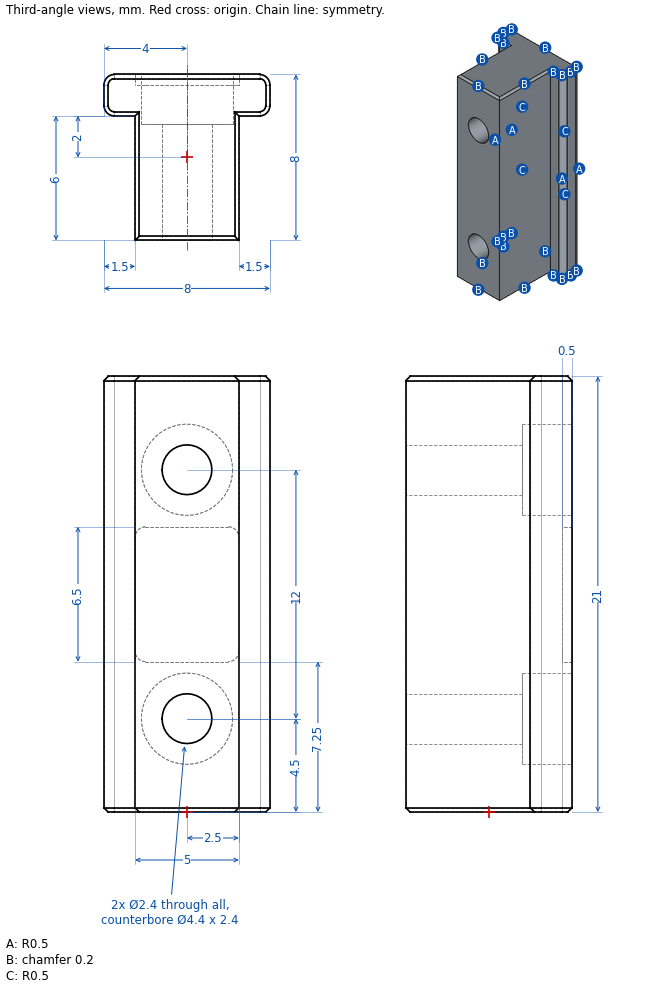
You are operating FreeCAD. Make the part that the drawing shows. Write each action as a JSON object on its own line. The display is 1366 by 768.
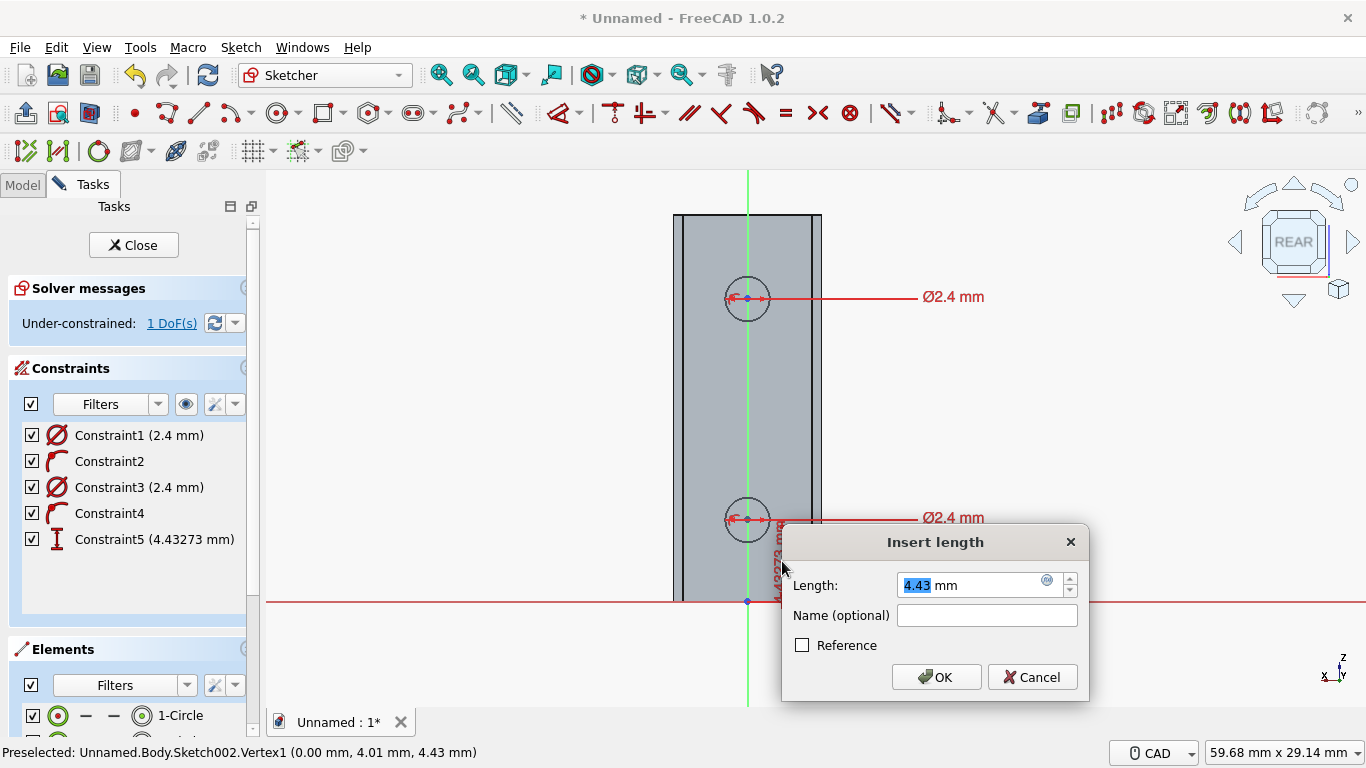
{"action": "type", "text": "4.5"}
{"action": "key", "text": "Return"}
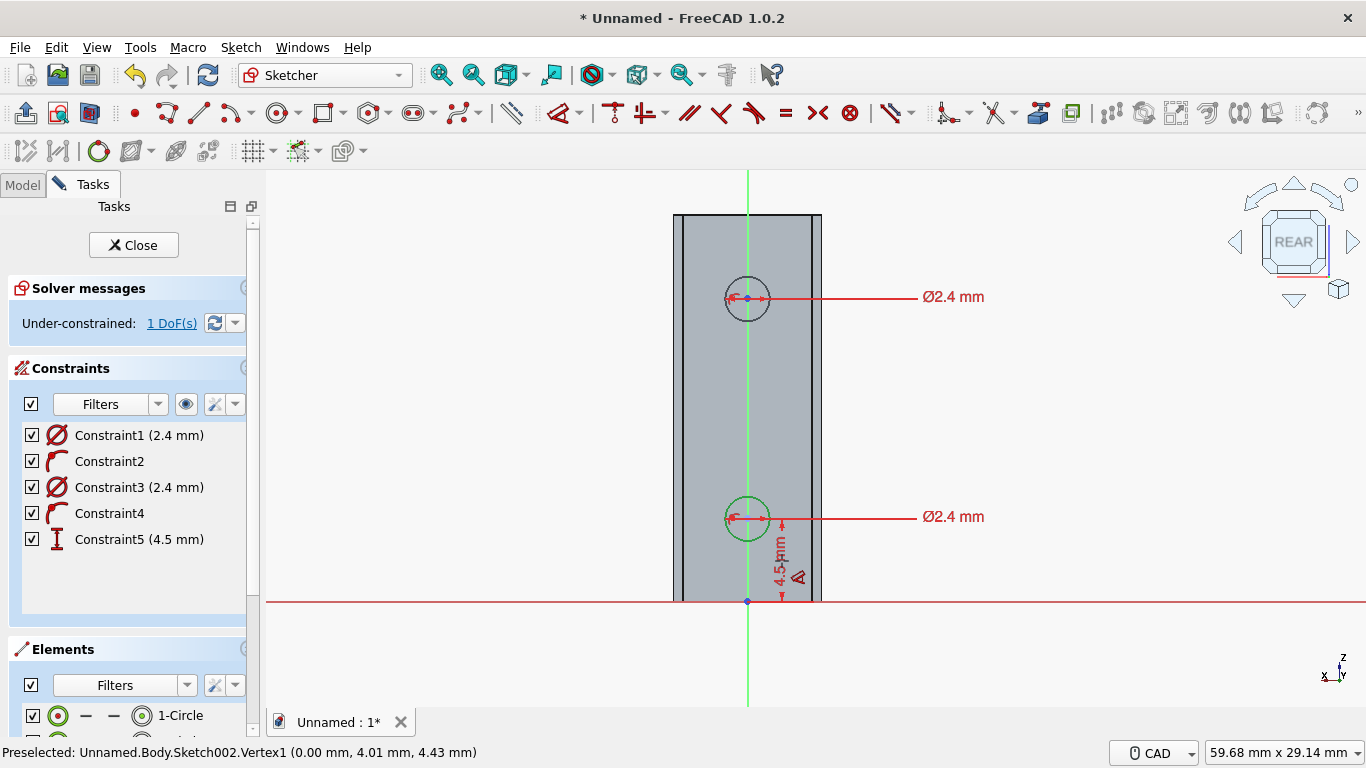
{"action": "left_click", "coordinate": [748, 519]}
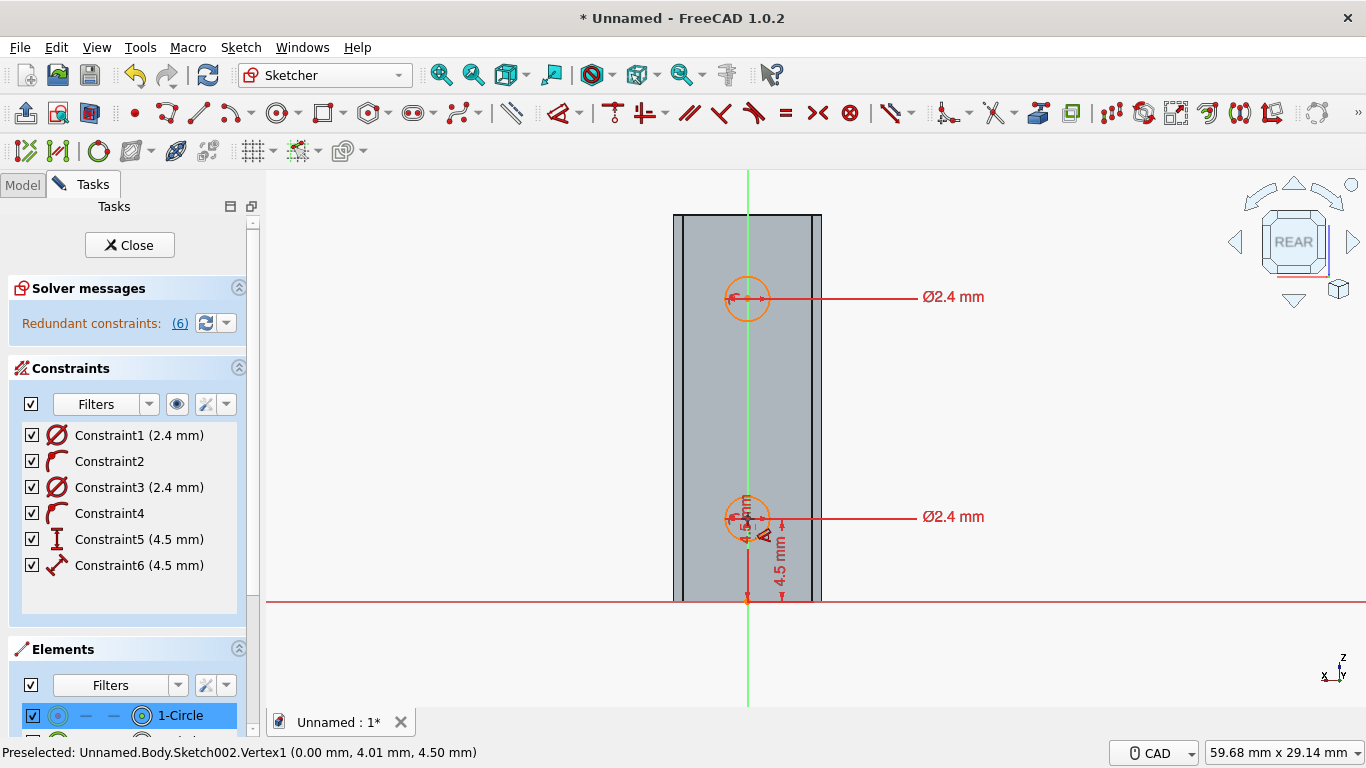
{"action": "left_click", "coordinate": [748, 299]}
{"action": "left_click", "coordinate": [782, 409]}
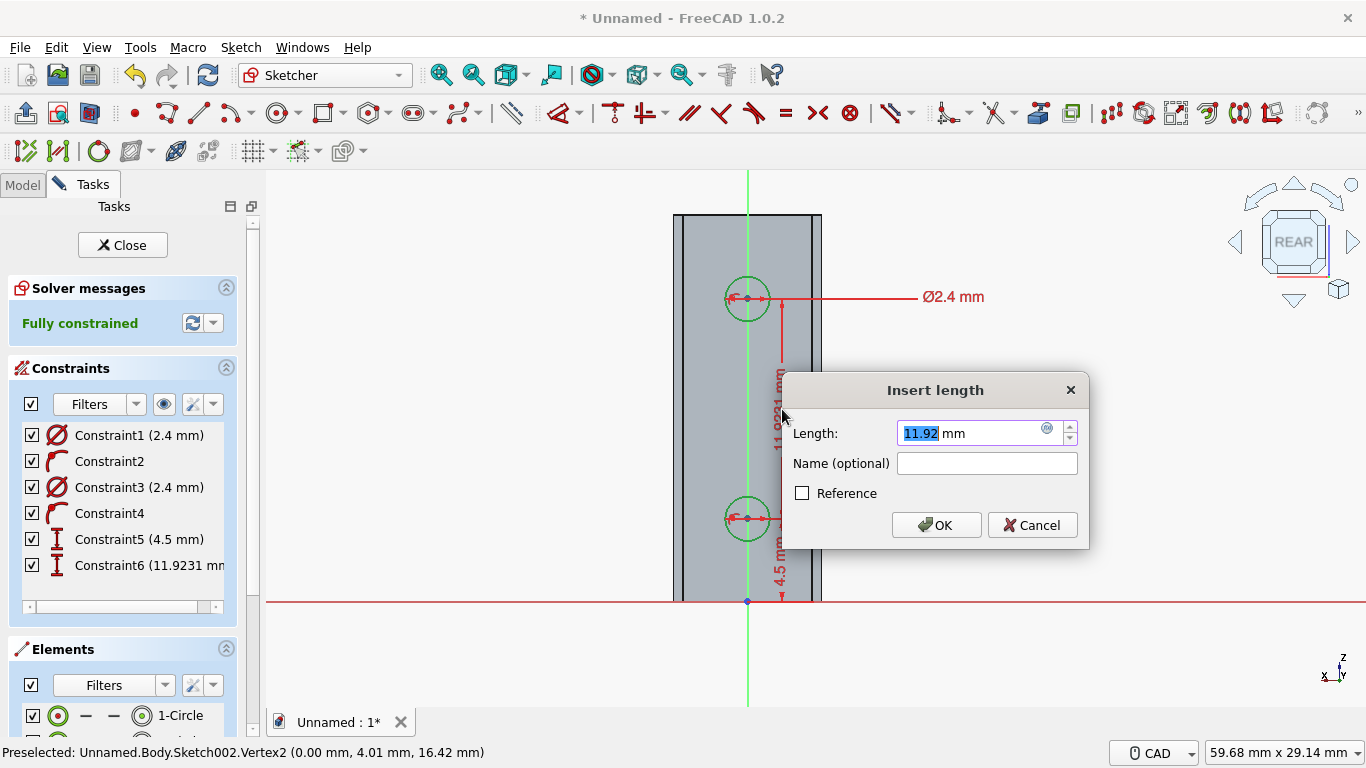
{"action": "type", "text": "12"}
{"action": "key", "text": "Return"}
{"action": "key", "text": "Escape"}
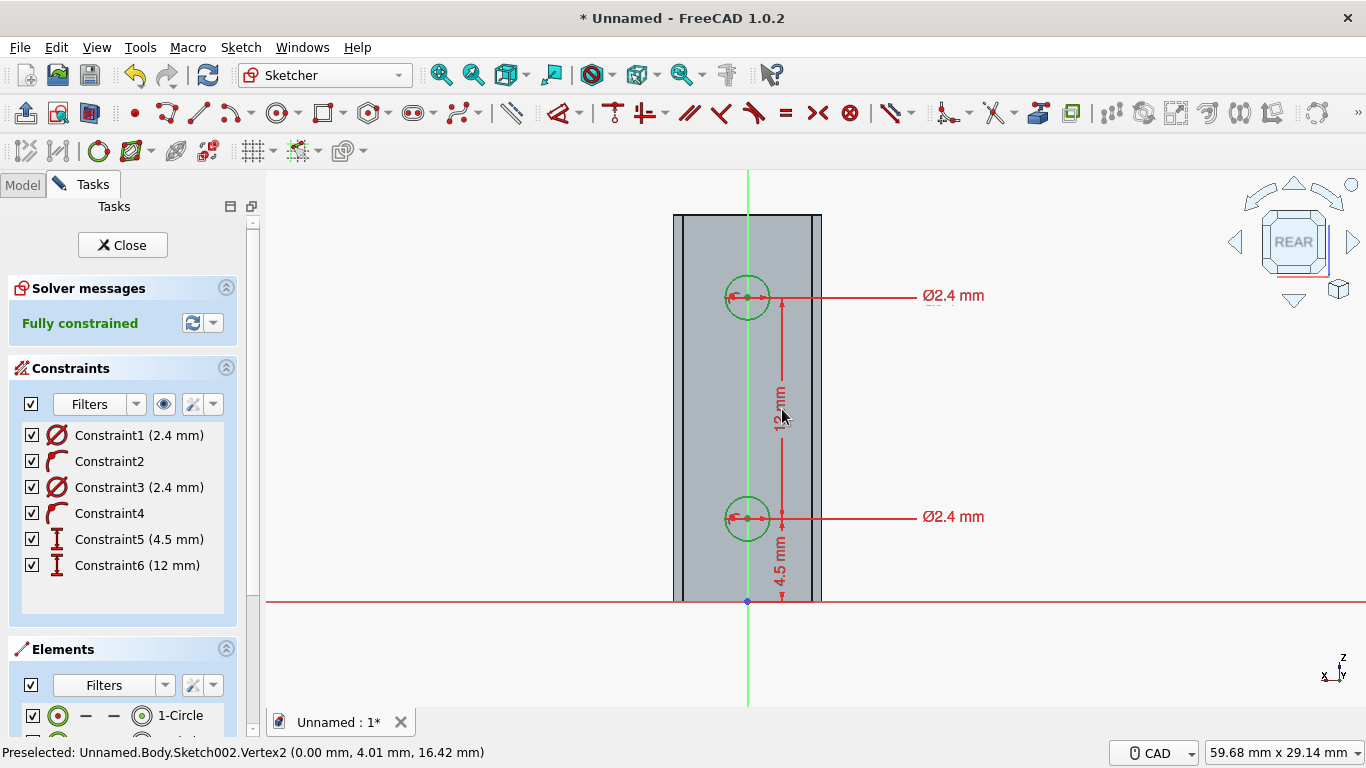
{"action": "left_click", "coordinate": [123, 245]}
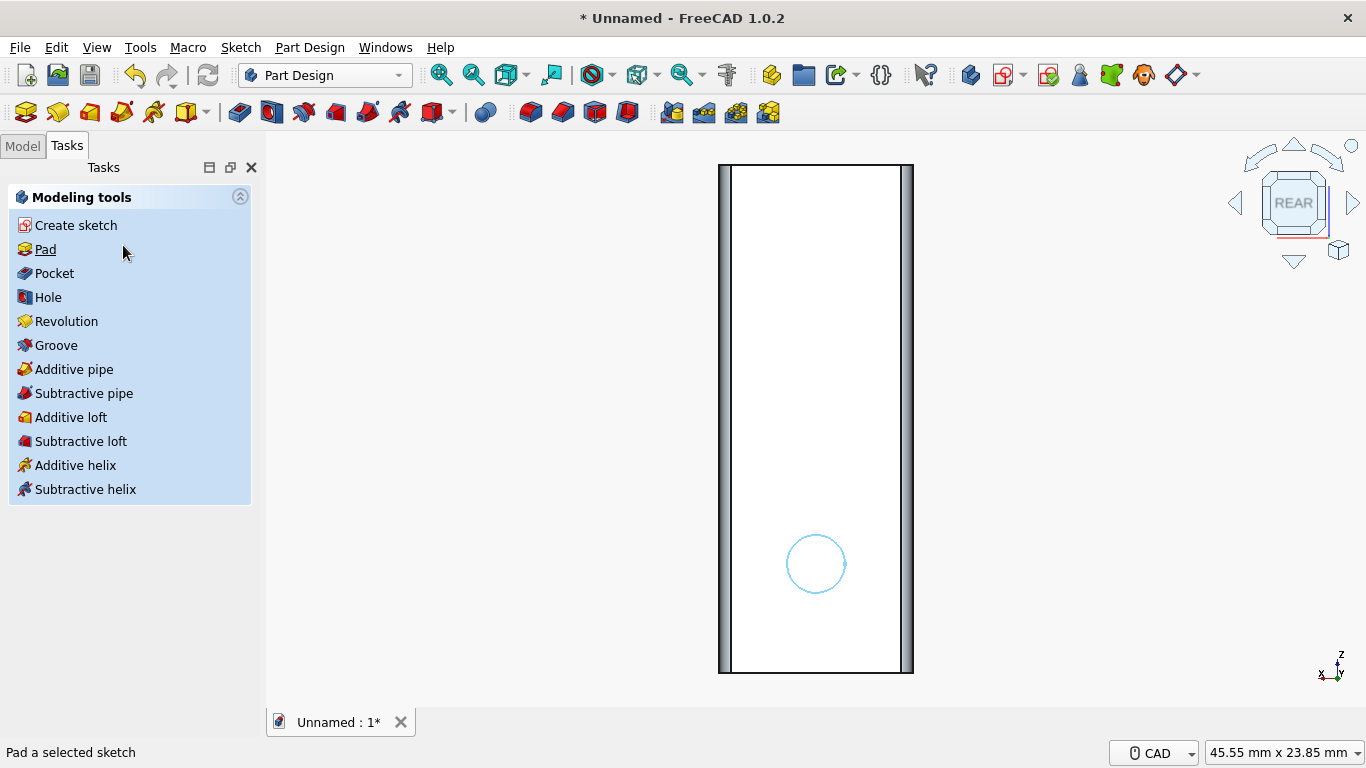
{"action": "left_click", "coordinate": [272, 112]}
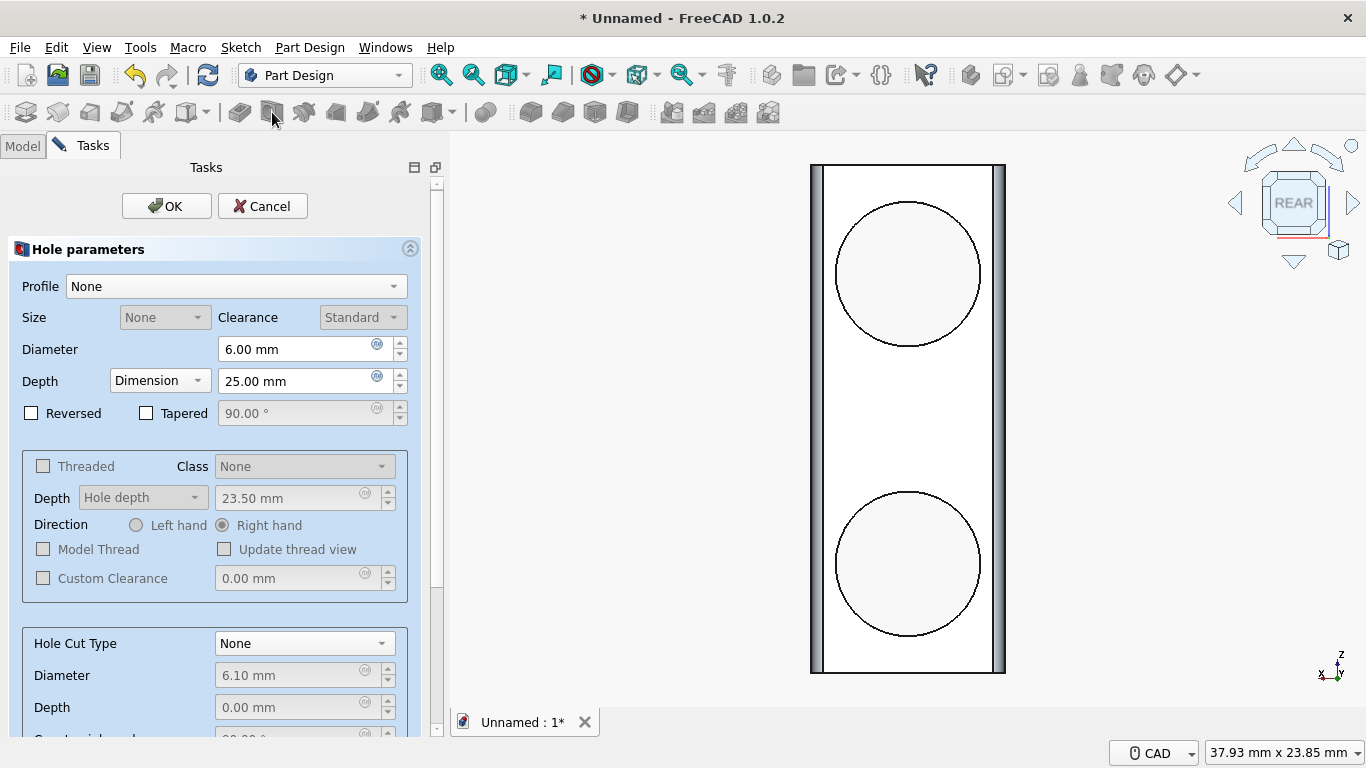
{"action": "triple_click", "coordinate": [305, 349]}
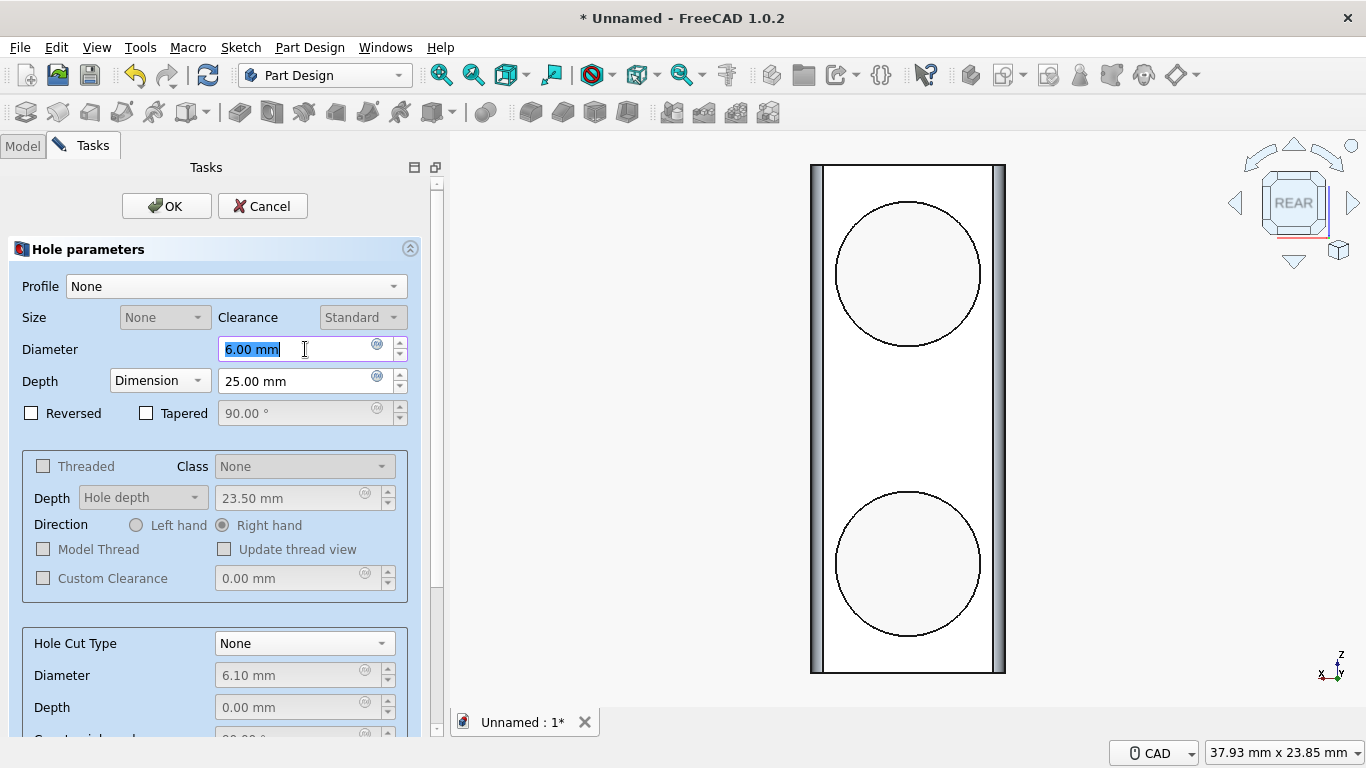
{"action": "type", "text": "2.4"}
{"action": "key", "text": "Tab"}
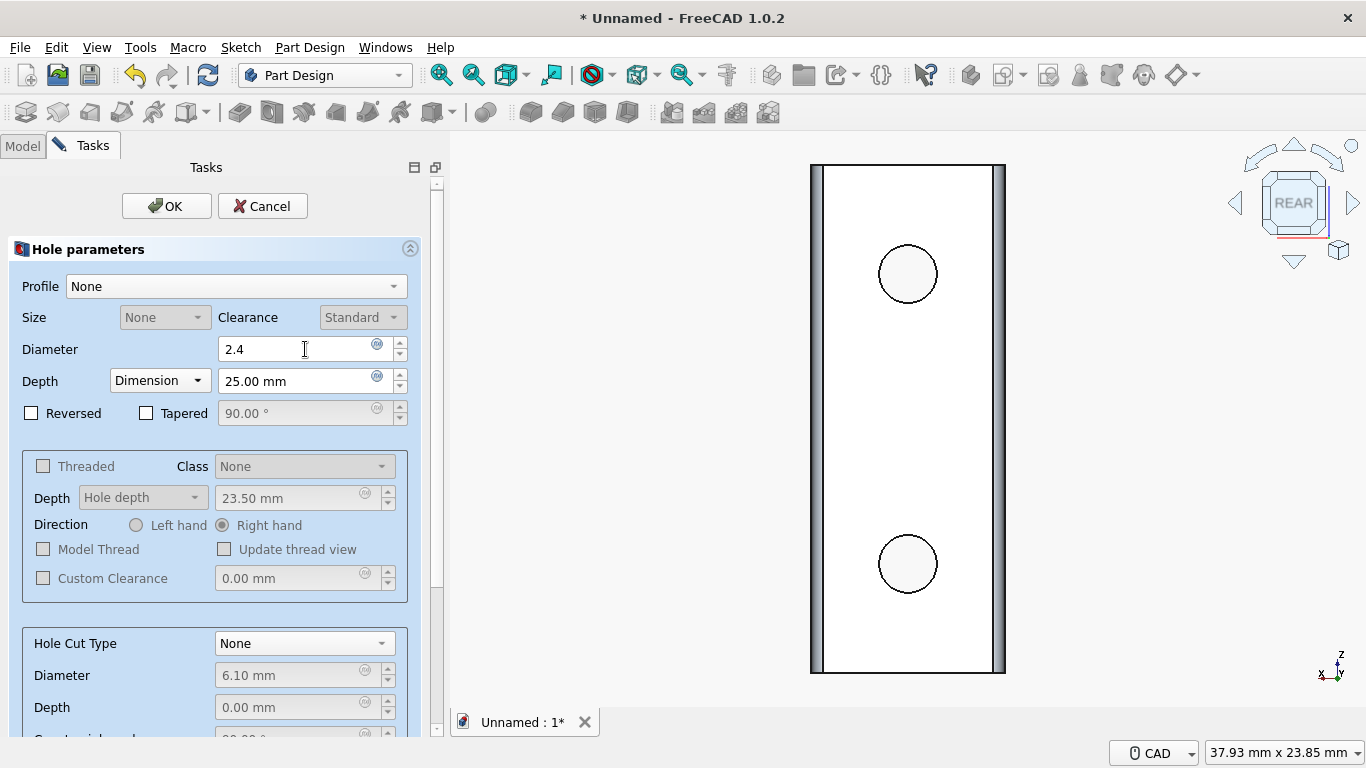
{"action": "left_click", "coordinate": [161, 380]}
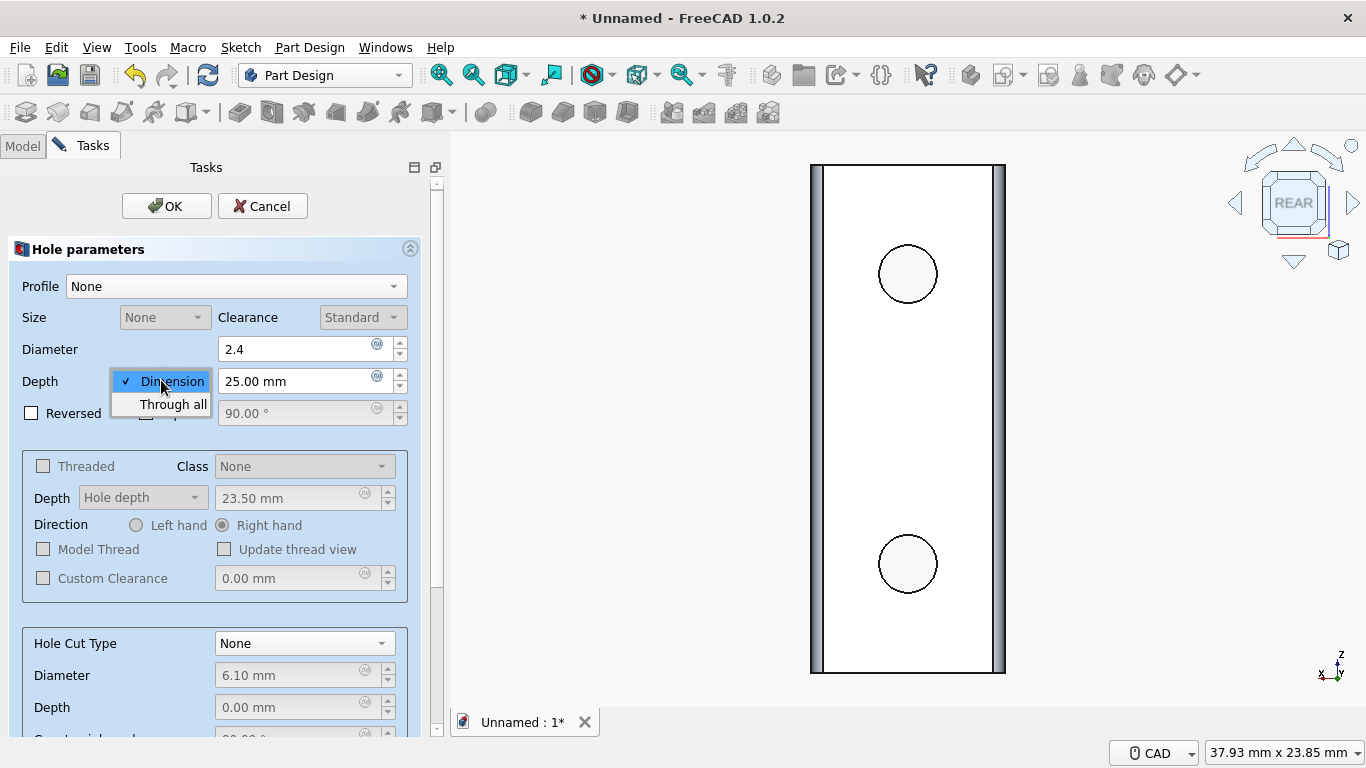
{"action": "left_click", "coordinate": [160, 404]}